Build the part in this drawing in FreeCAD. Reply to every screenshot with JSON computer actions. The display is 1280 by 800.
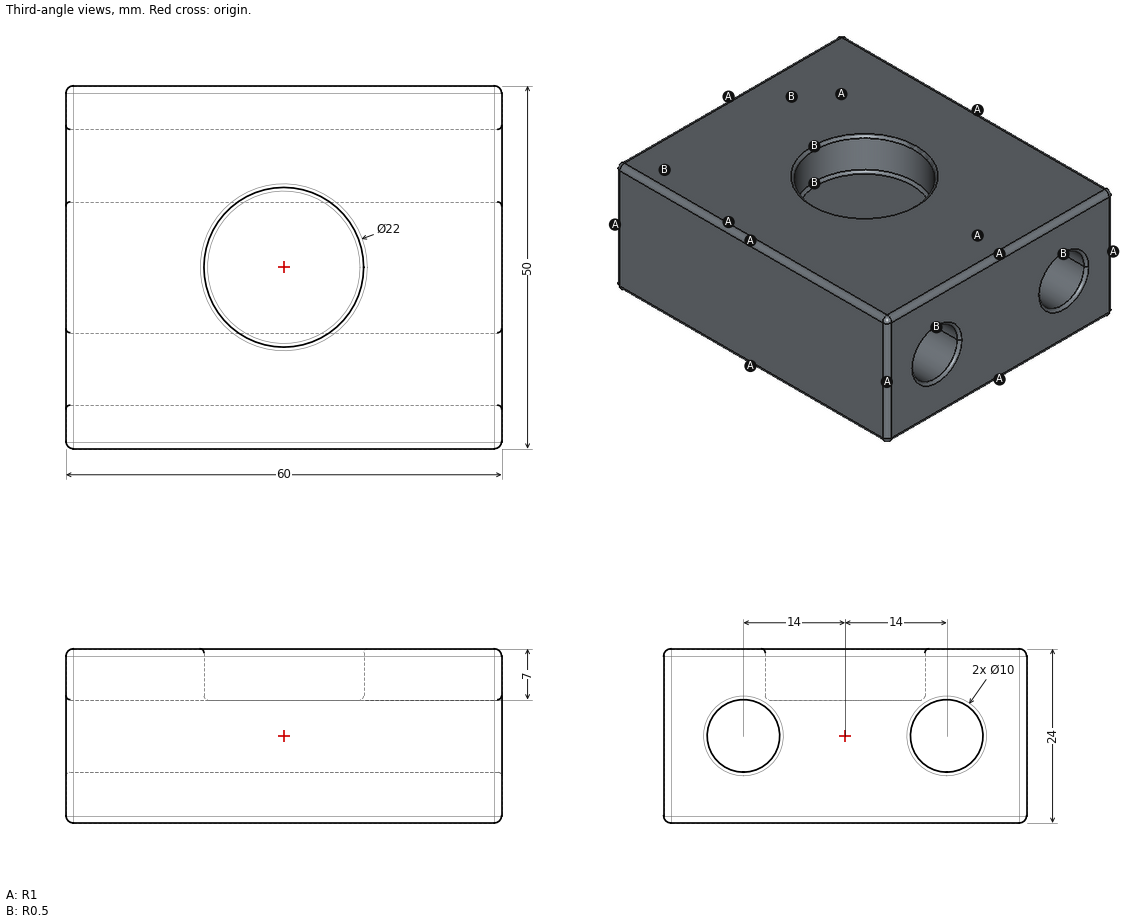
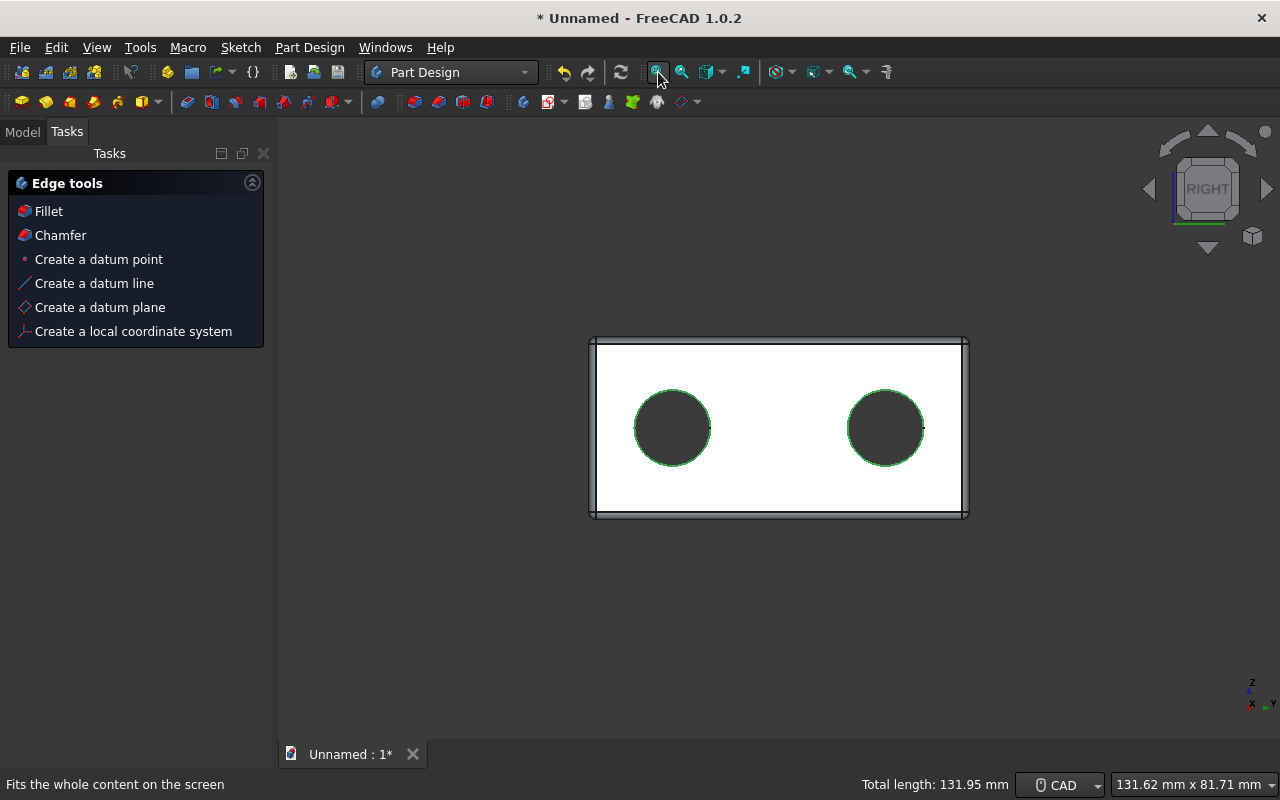
{"action": "key", "text": "5"}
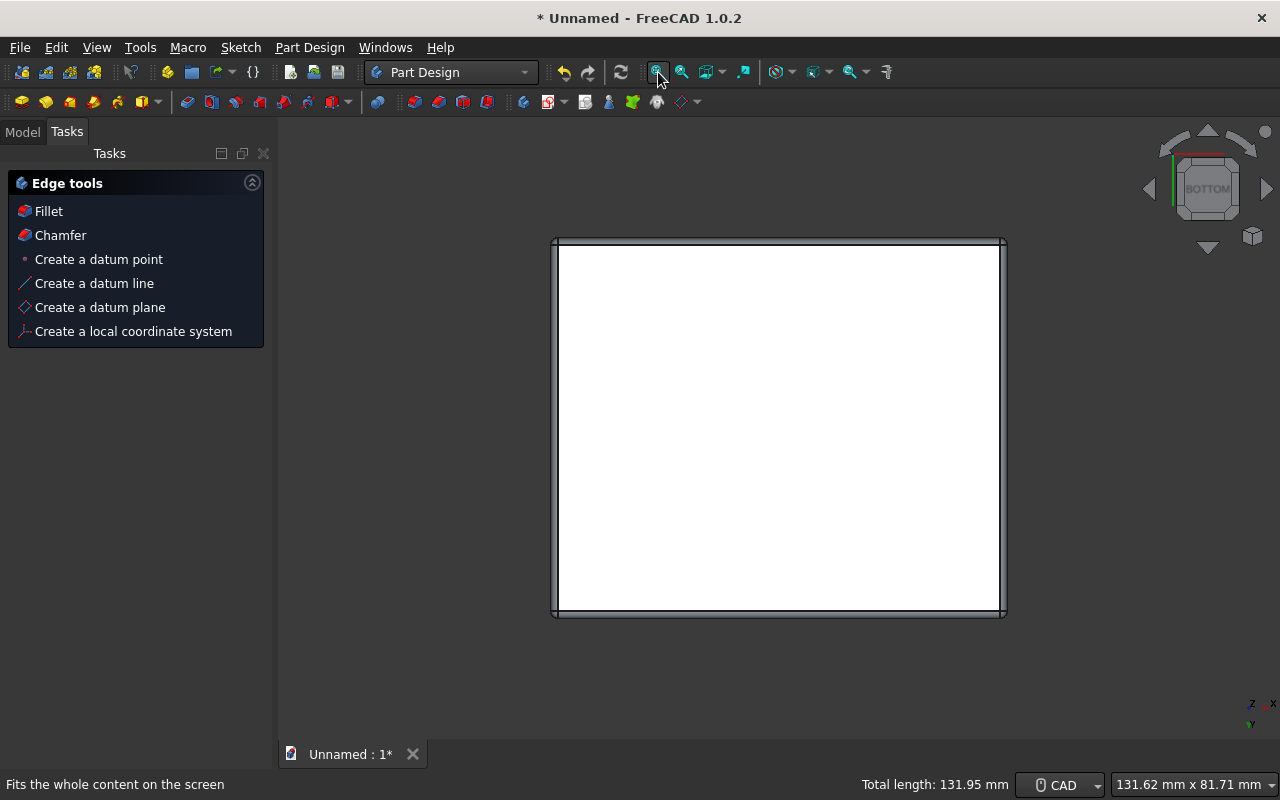
{"action": "key", "text": "4"}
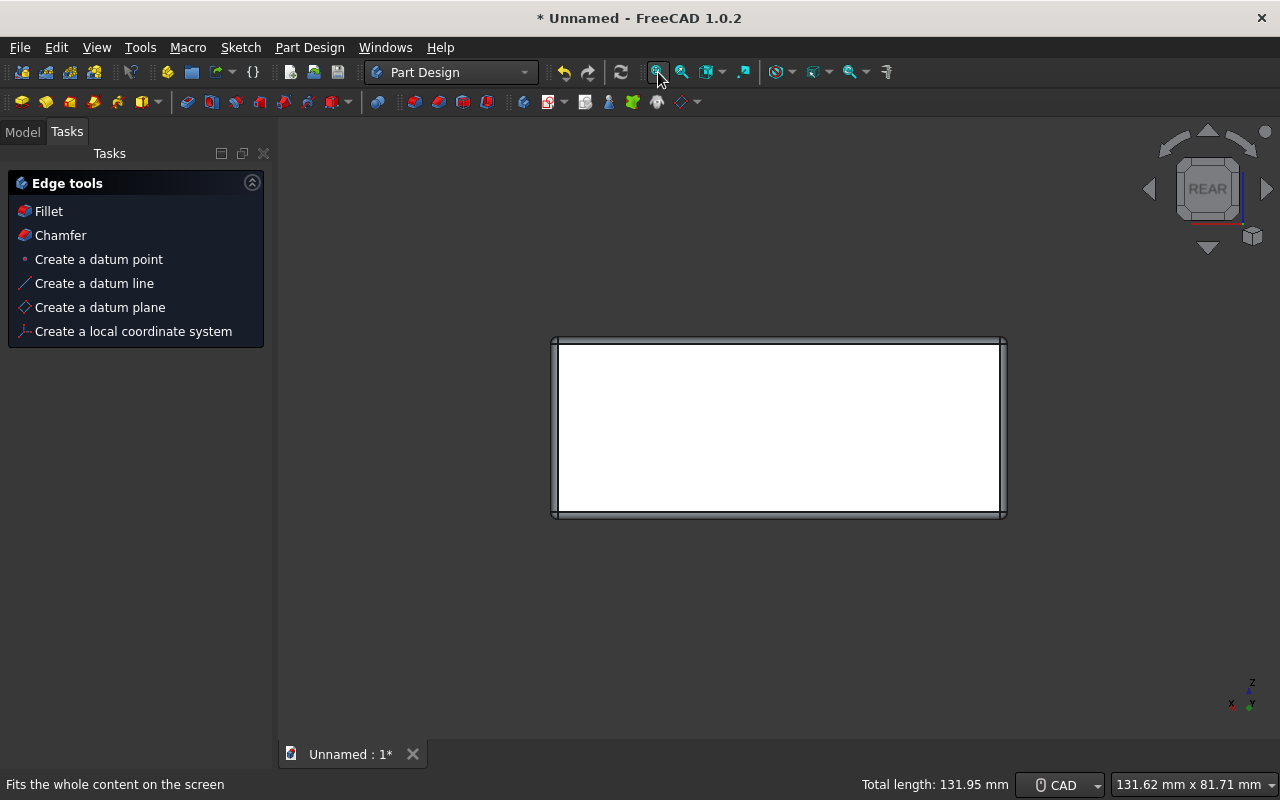
{"action": "key", "text": "6"}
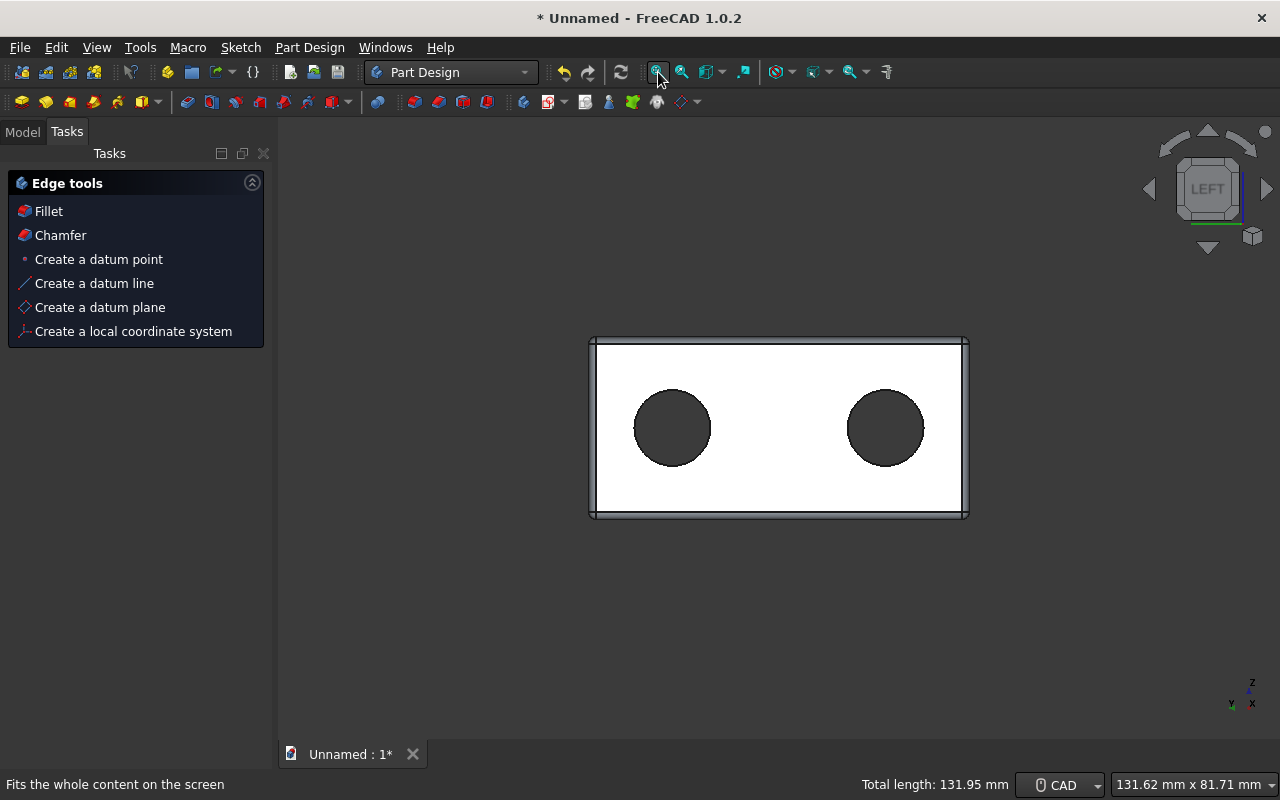
{"action": "left_click", "coordinate": [658, 72]}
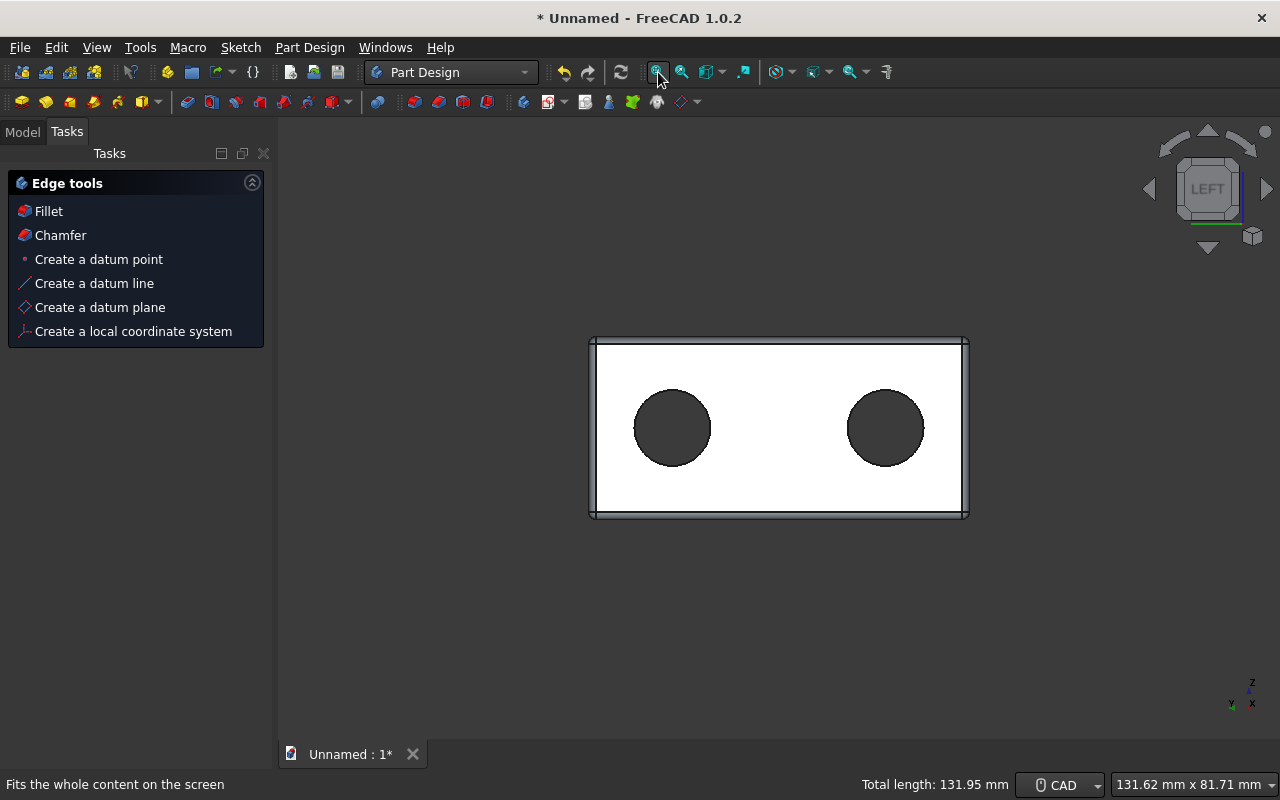
{"action": "left_click", "coordinate": [710, 427], "text": "ctrl"}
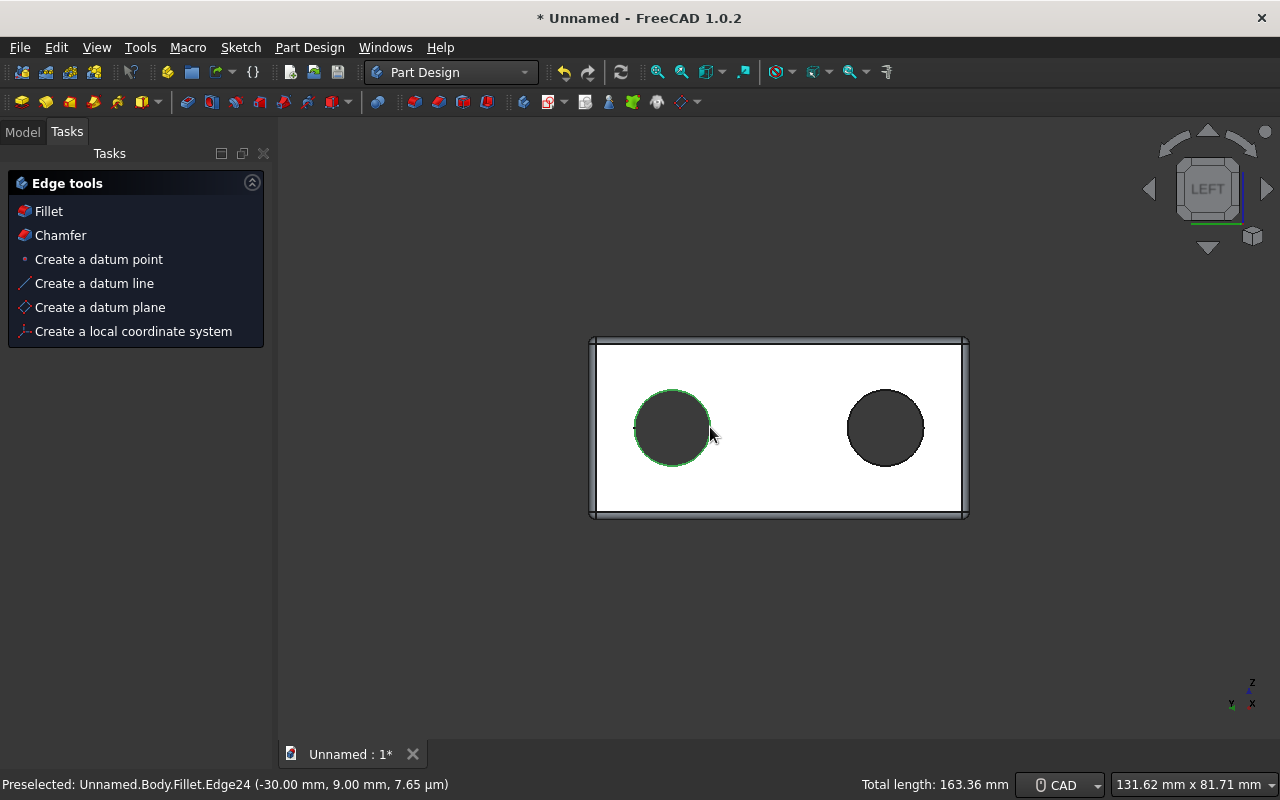
{"action": "left_click", "coordinate": [924, 427], "text": "ctrl"}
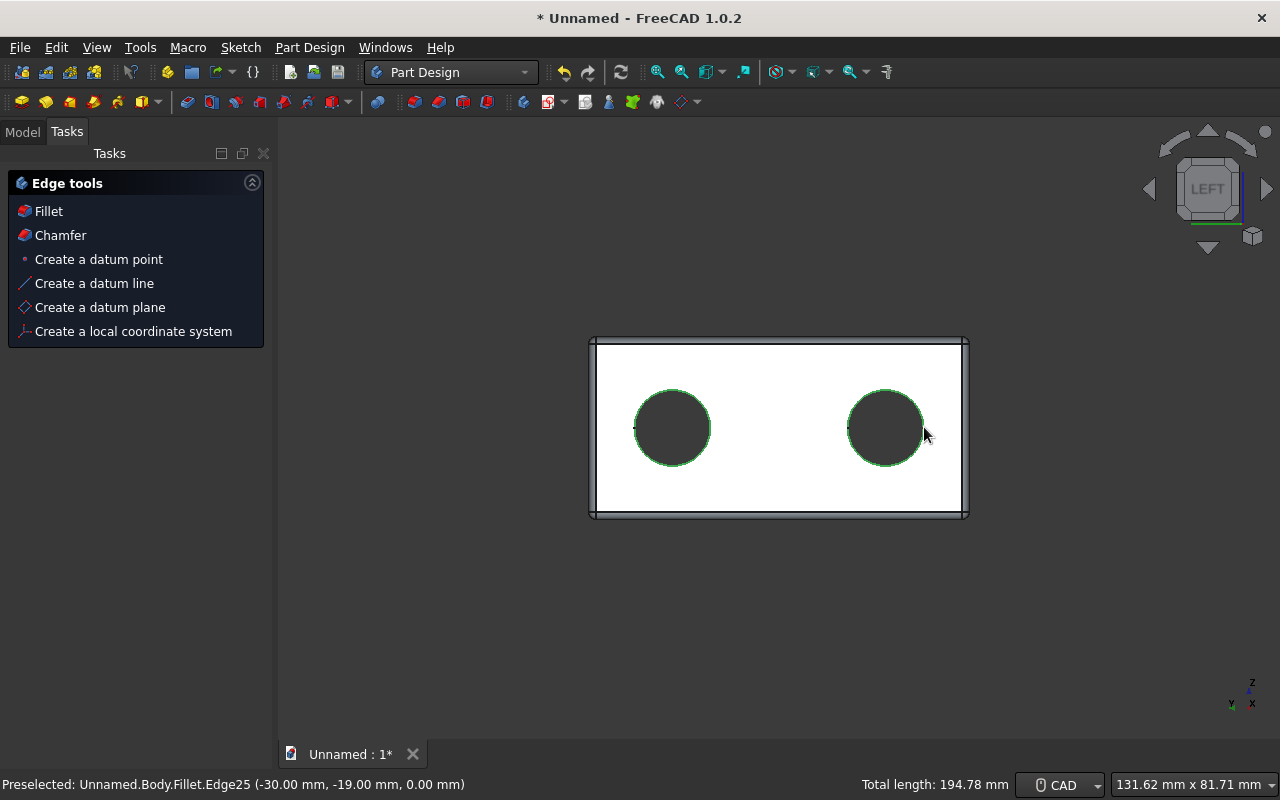
{"action": "key", "text": "v 3"}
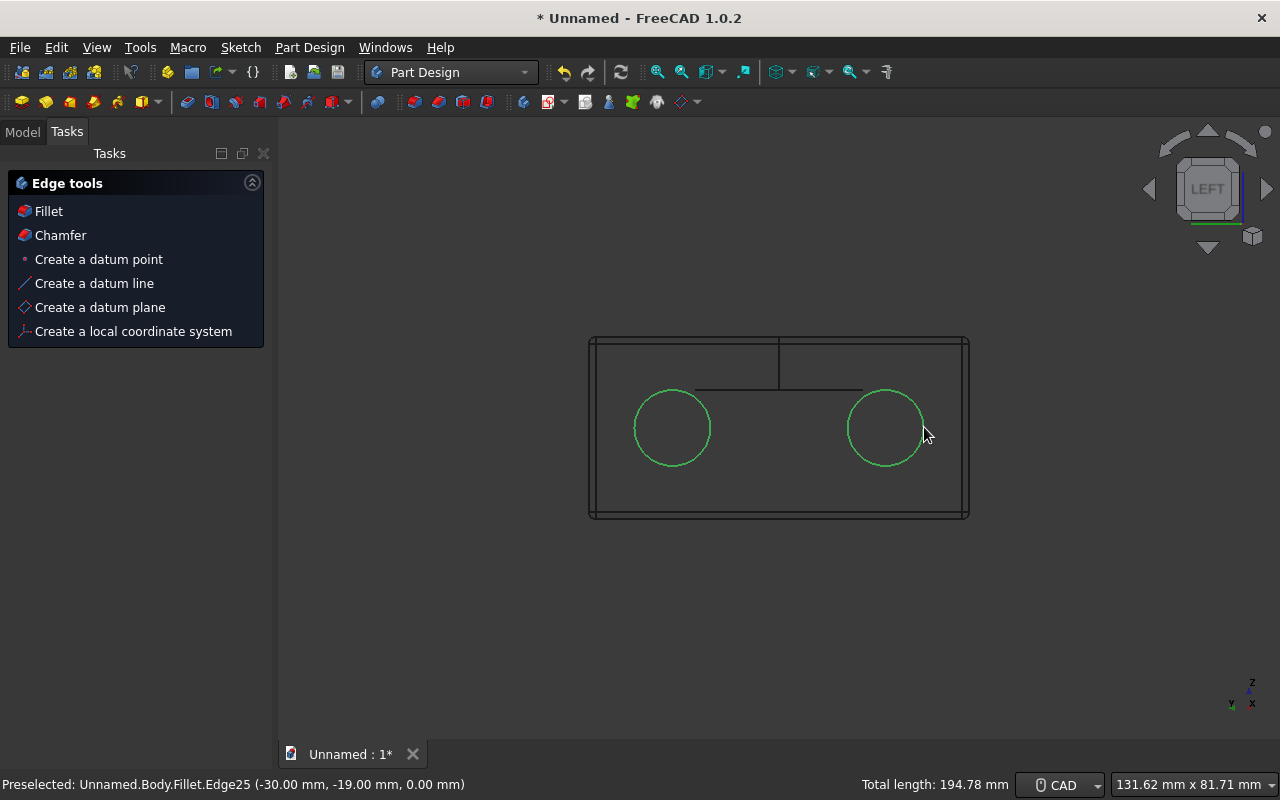
{"action": "key", "text": "0"}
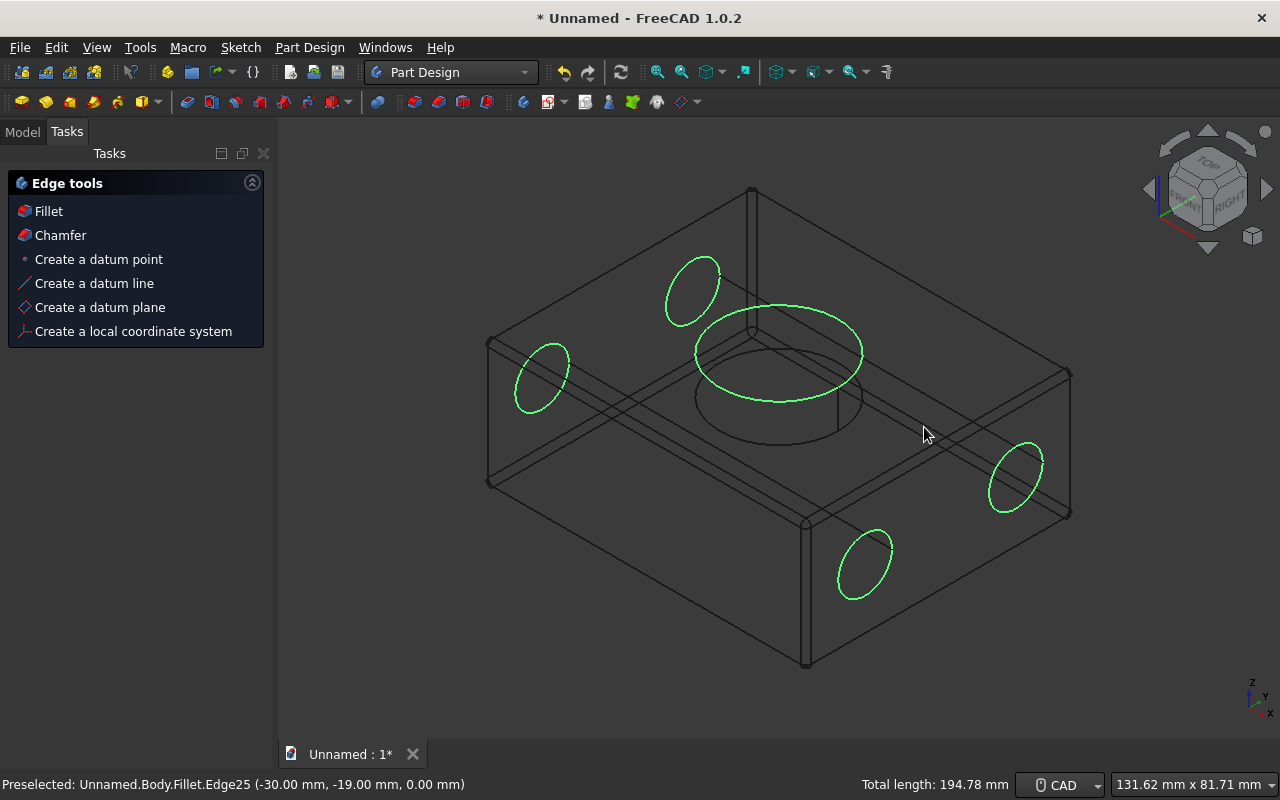
{"action": "left_click", "coordinate": [720, 362], "text": "ctrl"}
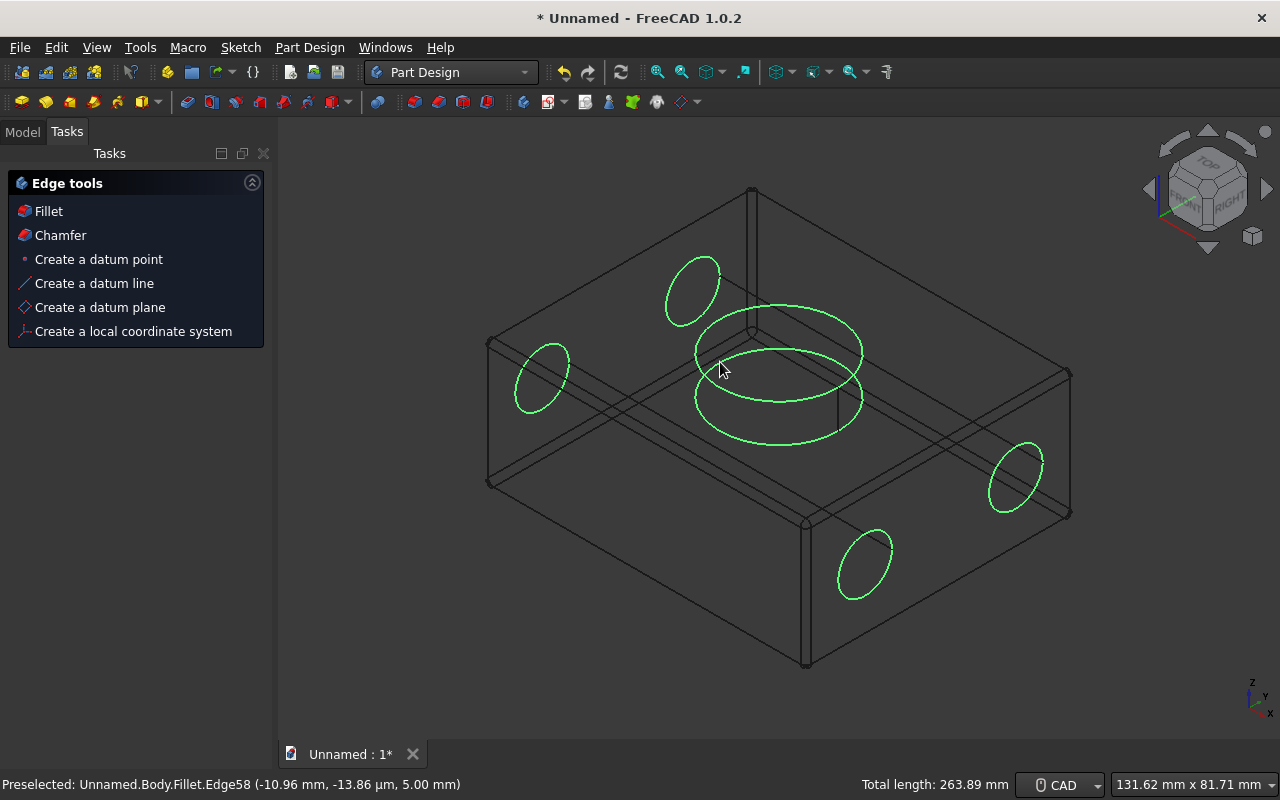
{"action": "key", "text": "v 1"}